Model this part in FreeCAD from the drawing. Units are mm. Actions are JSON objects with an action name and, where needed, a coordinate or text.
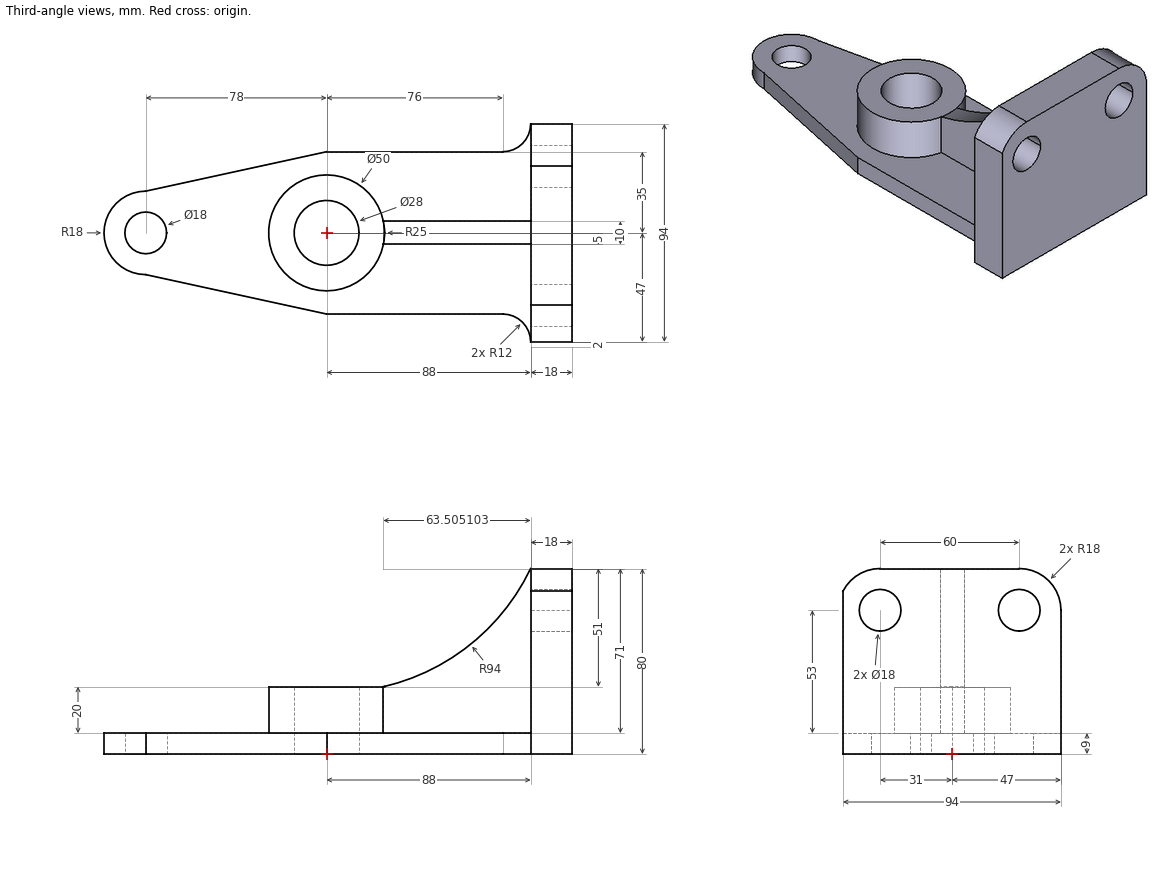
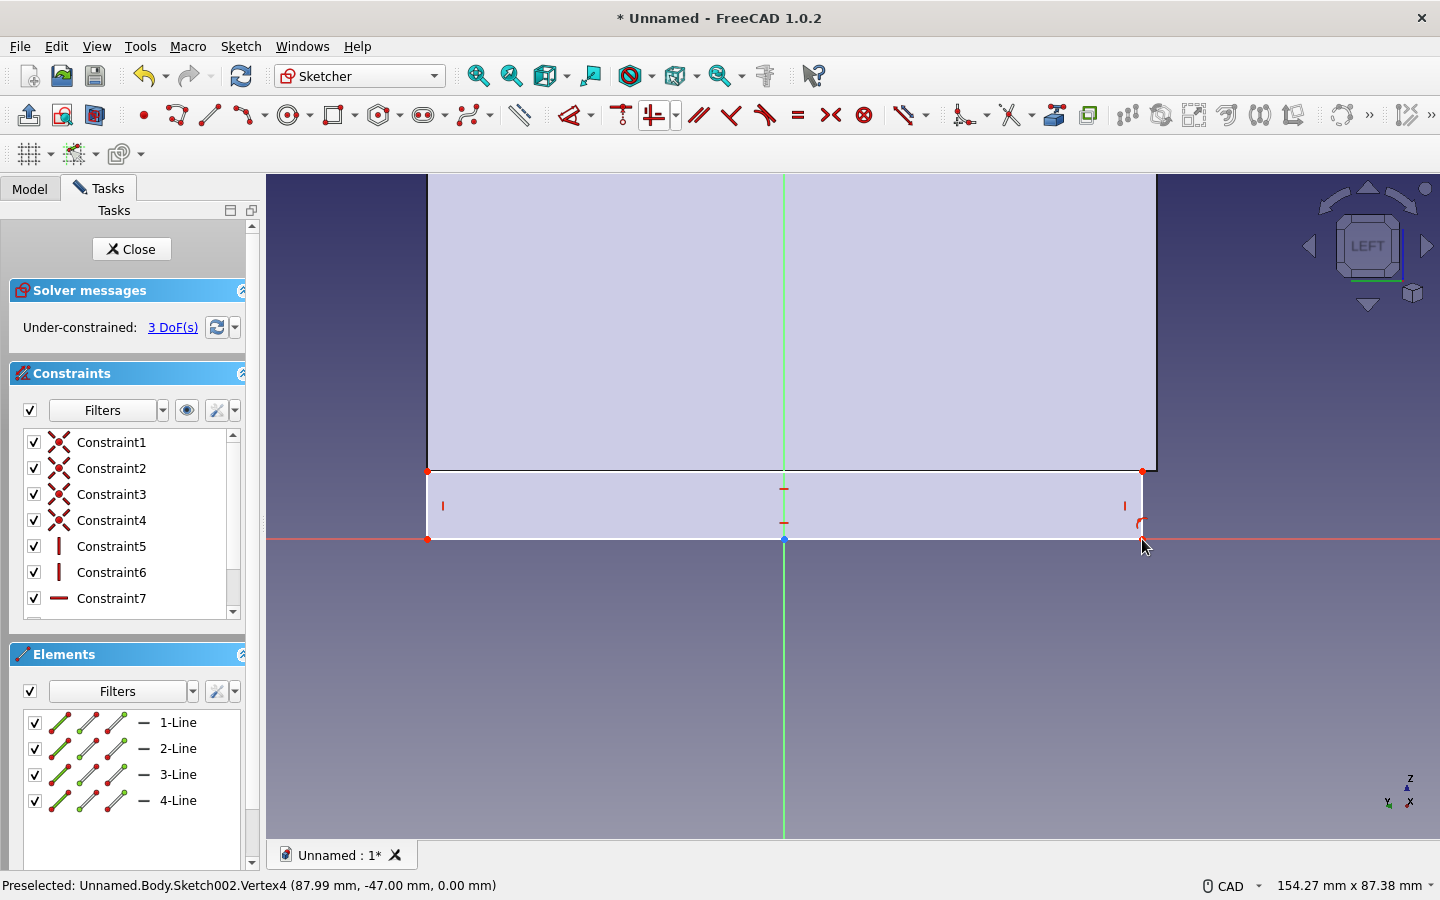
{"action": "key", "text": "d"}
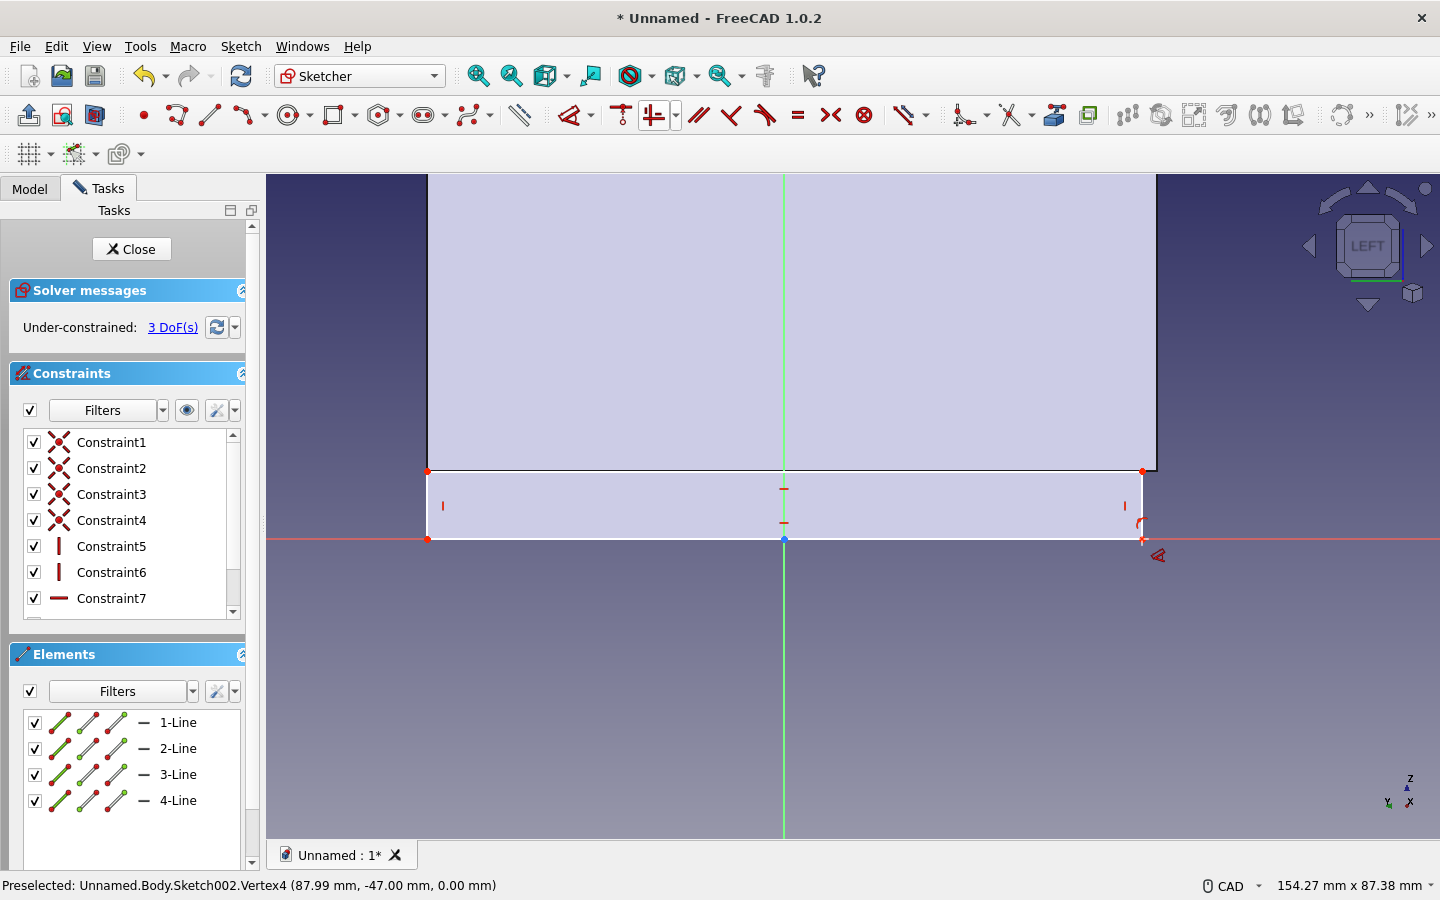
{"action": "left_click", "coordinate": [427, 492]}
{"action": "left_click", "coordinate": [393, 506]}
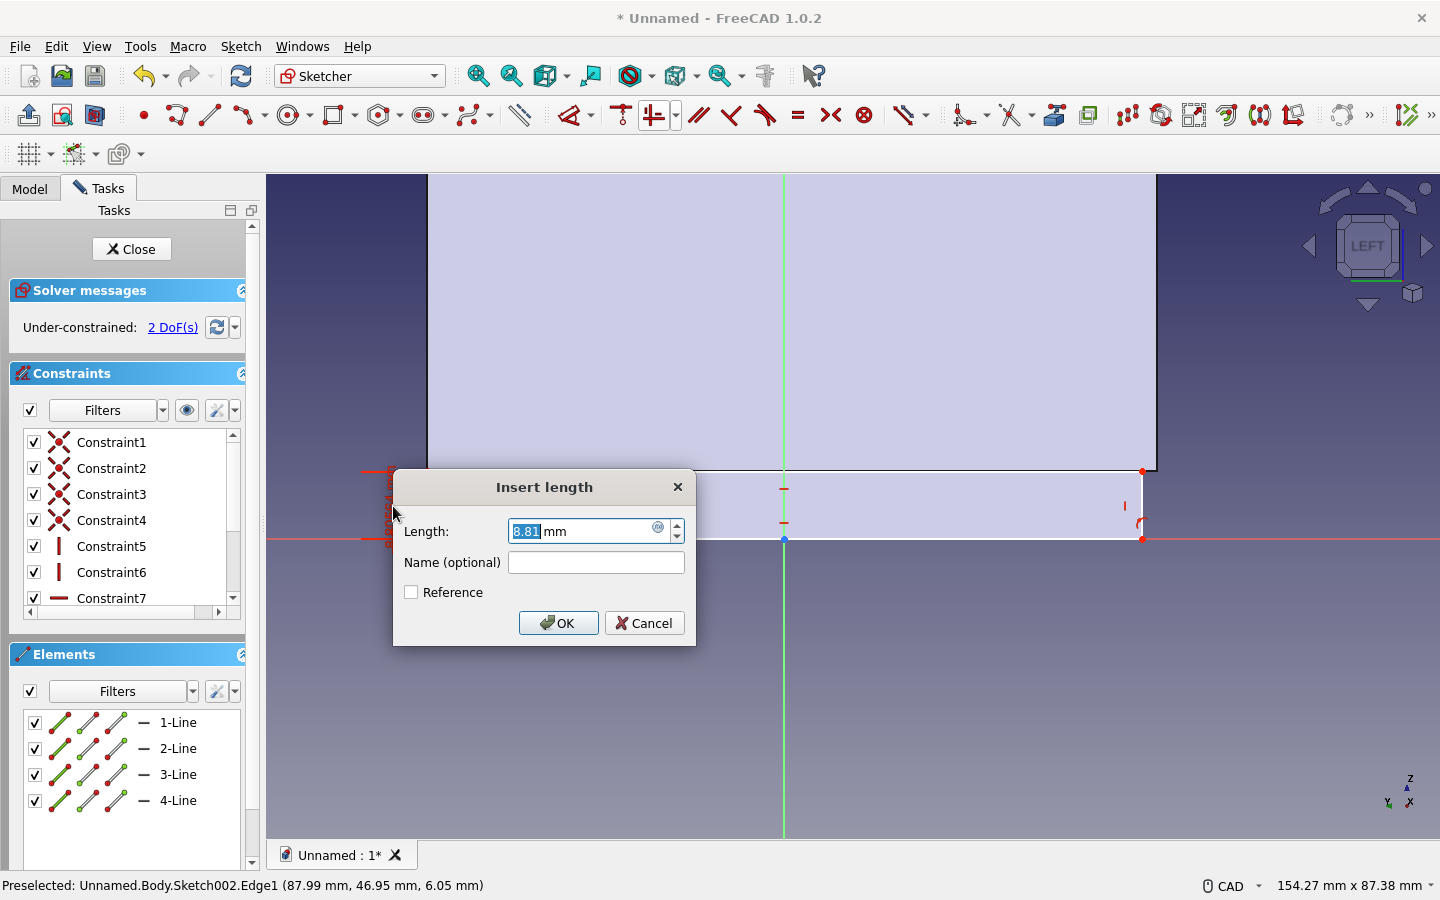
{"action": "type", "text": "9"}
{"action": "key", "text": "Return"}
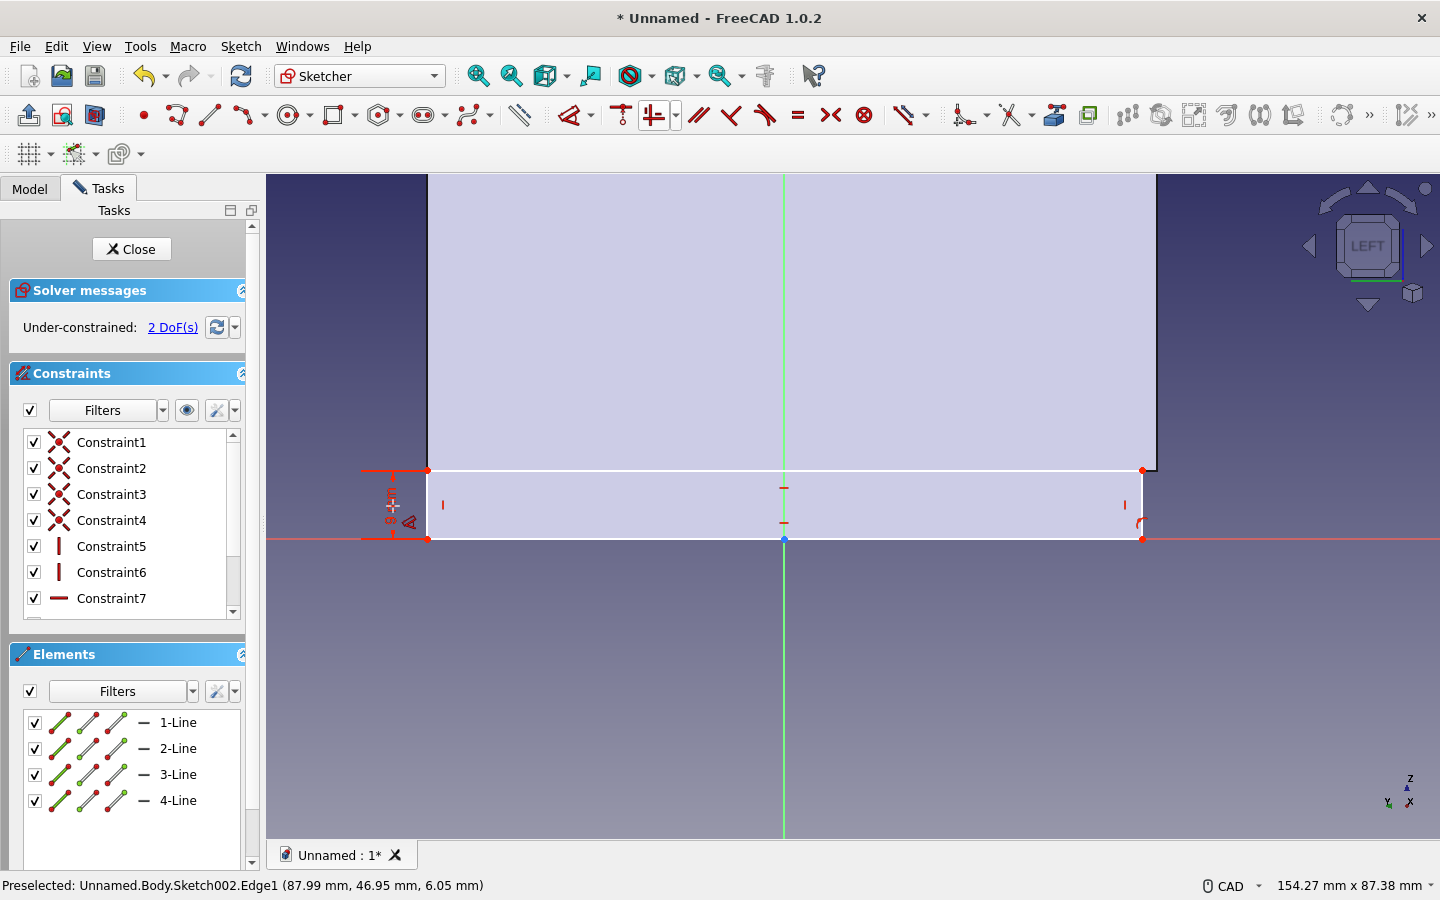
{"action": "left_click", "coordinate": [642, 539]}
{"action": "left_click", "coordinate": [620, 573]}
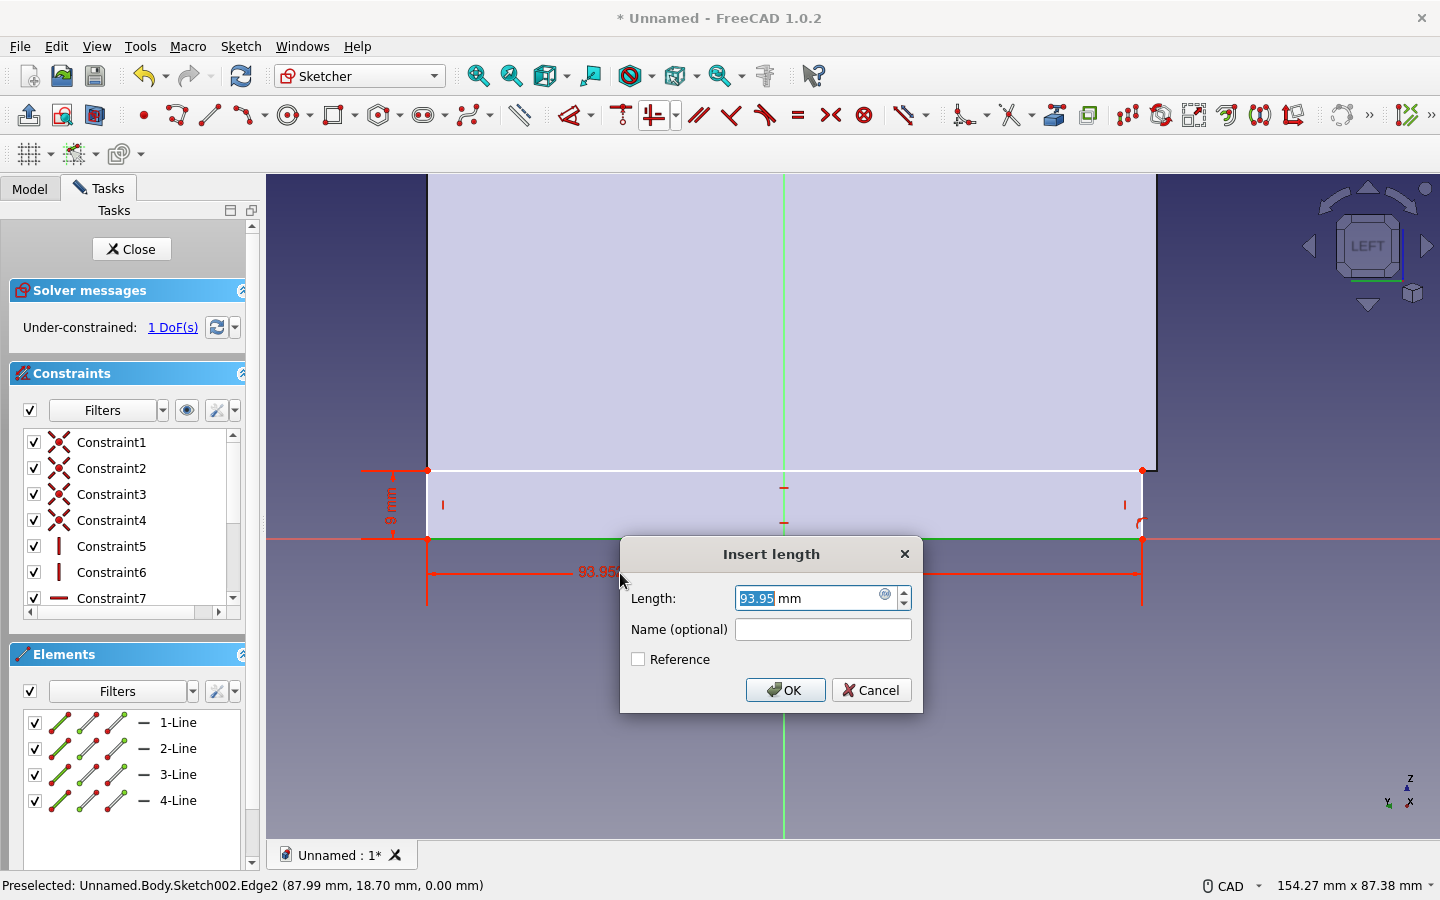
{"action": "type", "text": "94"}
{"action": "key", "text": "Return"}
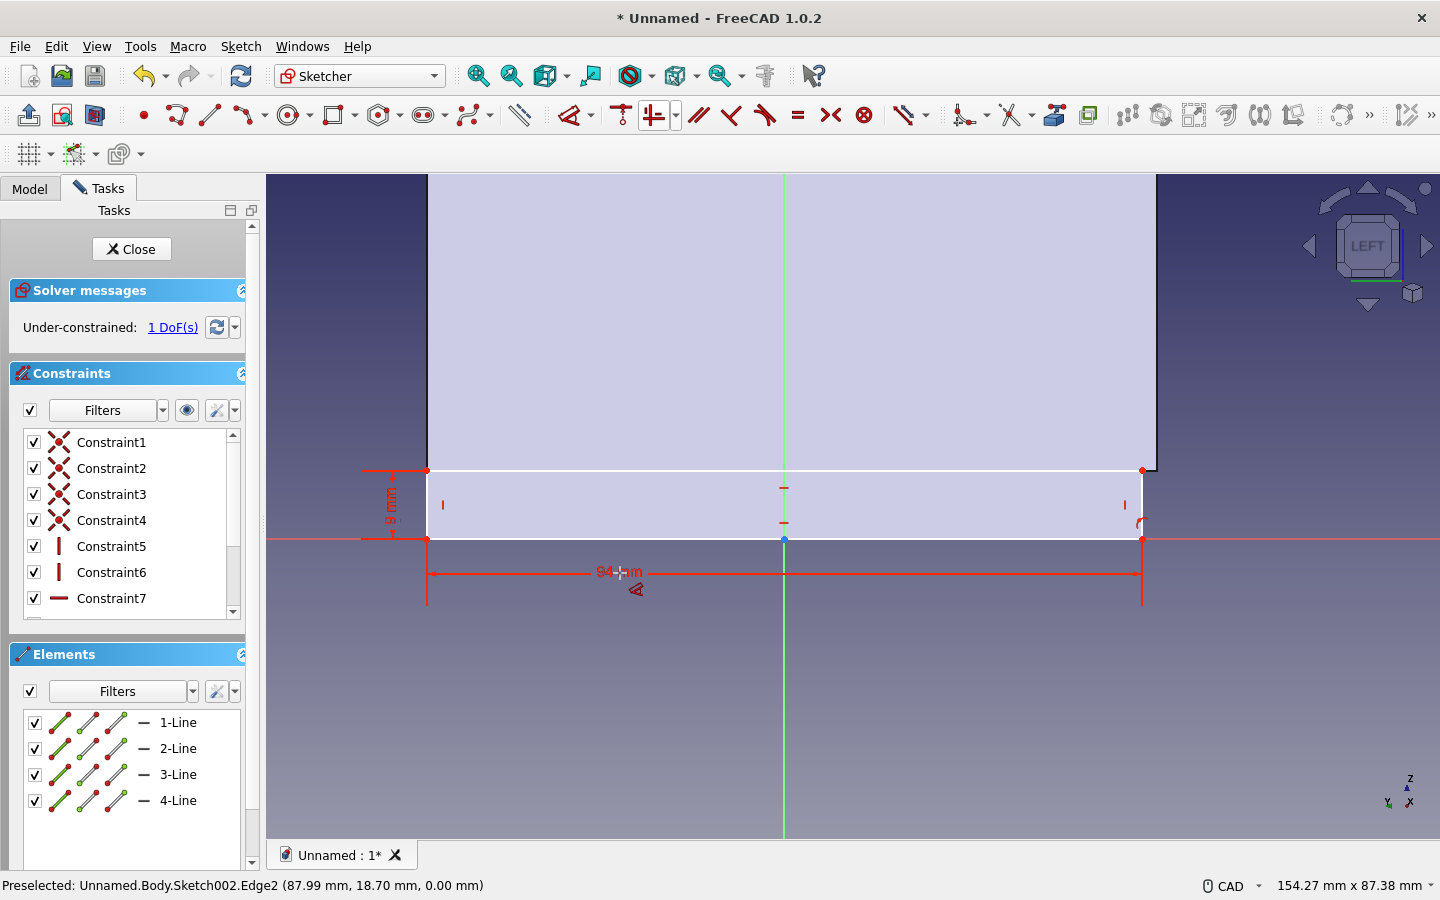
{"action": "left_click", "coordinate": [427, 471]}
{"action": "left_click", "coordinate": [523, 573]}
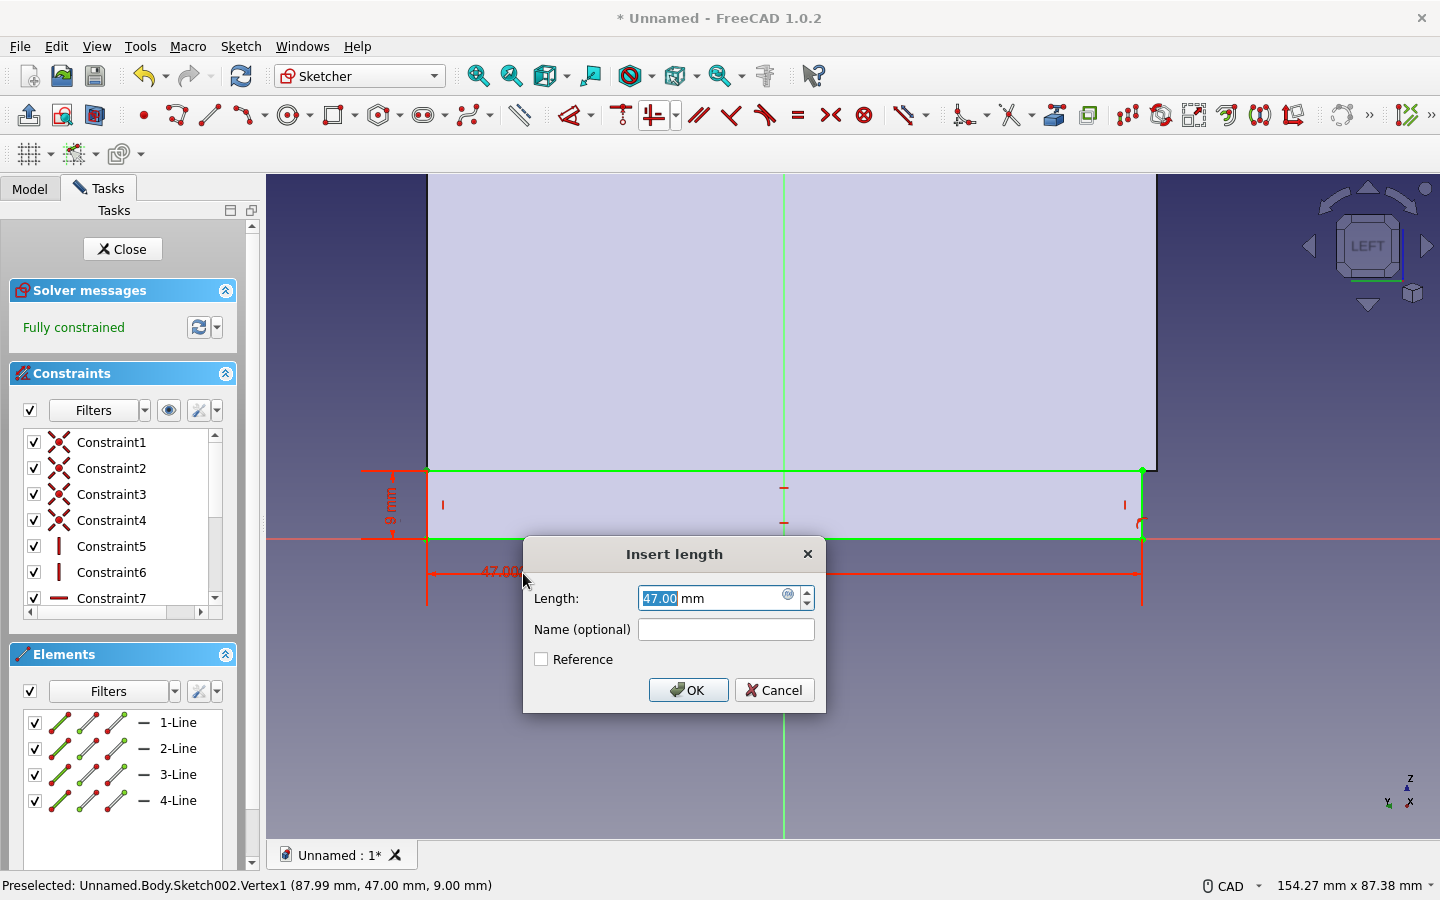
{"action": "type", "text": "47"}
{"action": "key", "text": "Return"}
{"action": "key", "text": "Escape"}